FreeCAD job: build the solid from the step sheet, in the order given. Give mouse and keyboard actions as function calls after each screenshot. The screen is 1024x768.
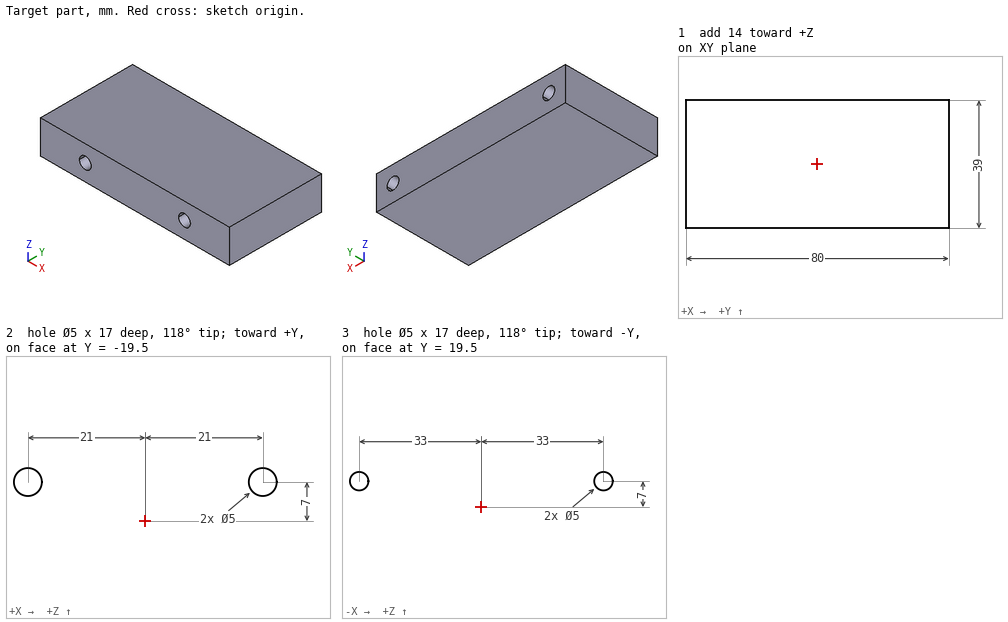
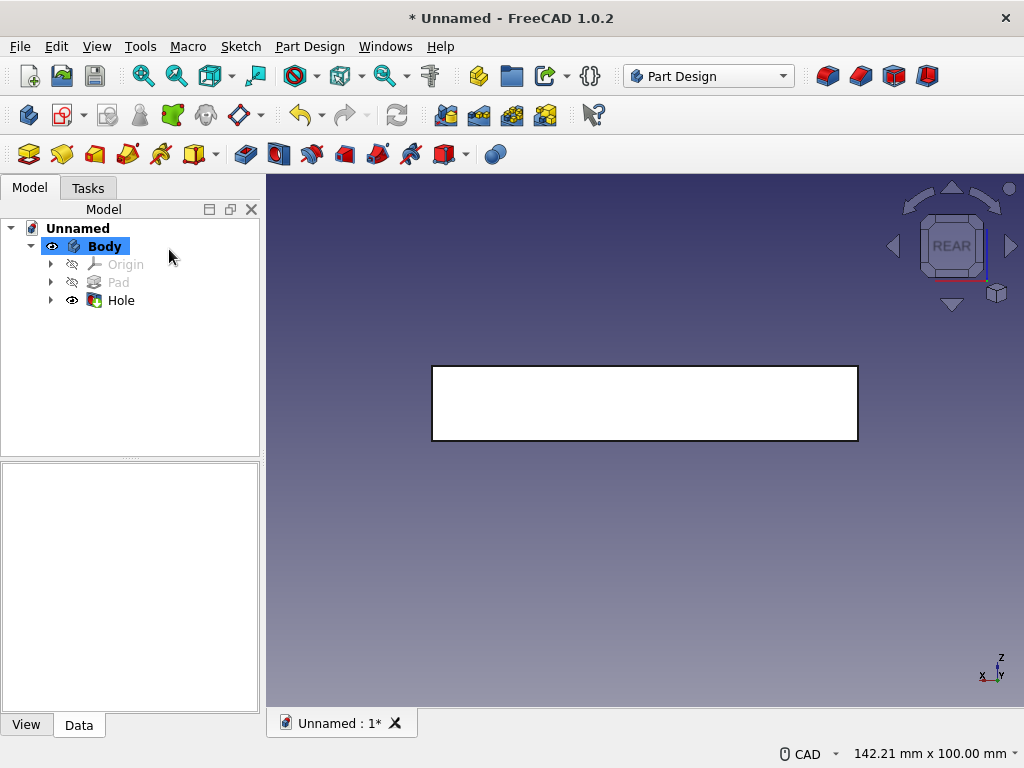
click(523, 402)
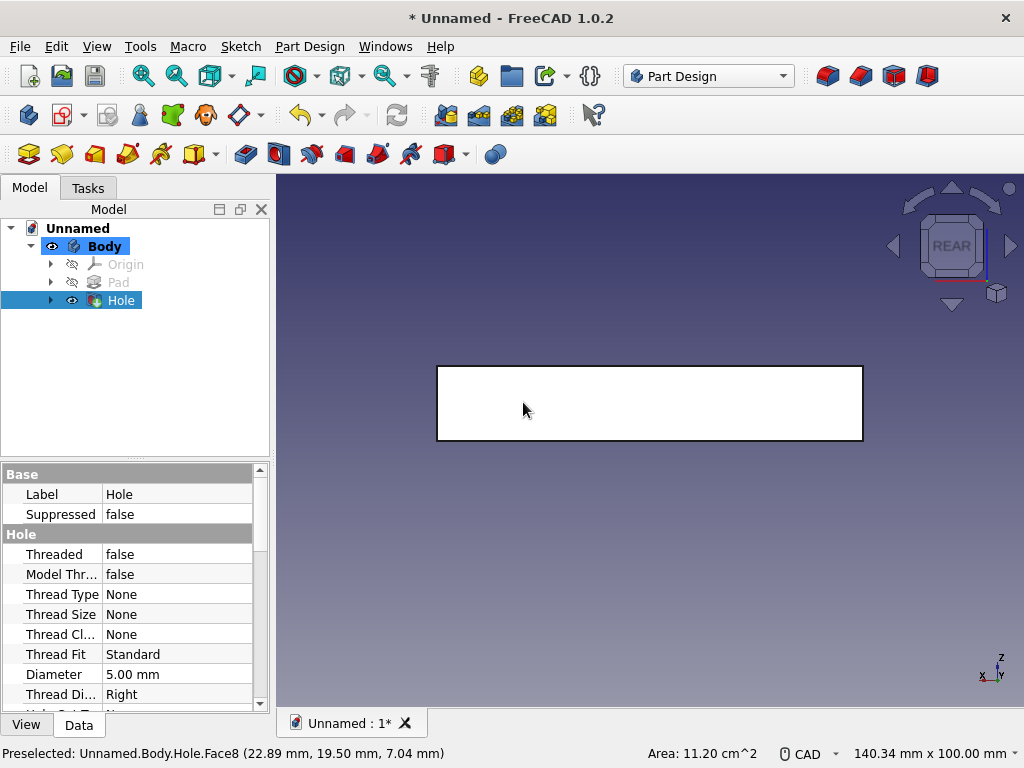
click(62, 116)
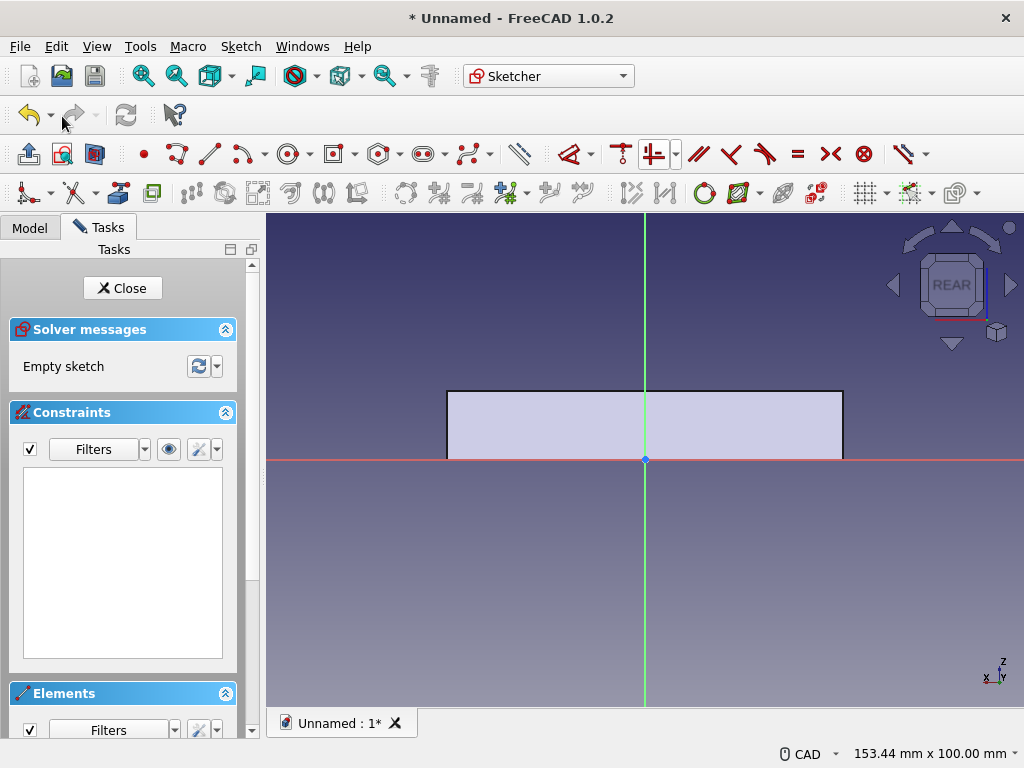
click(288, 154)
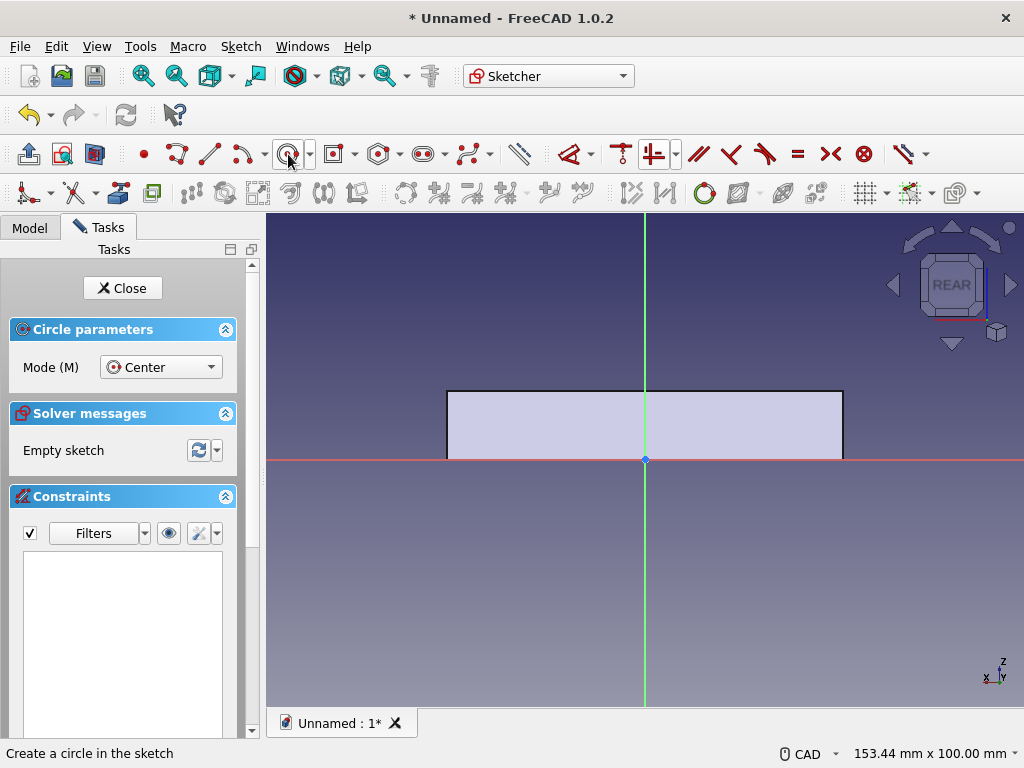
scroll(808, 425, up, 4)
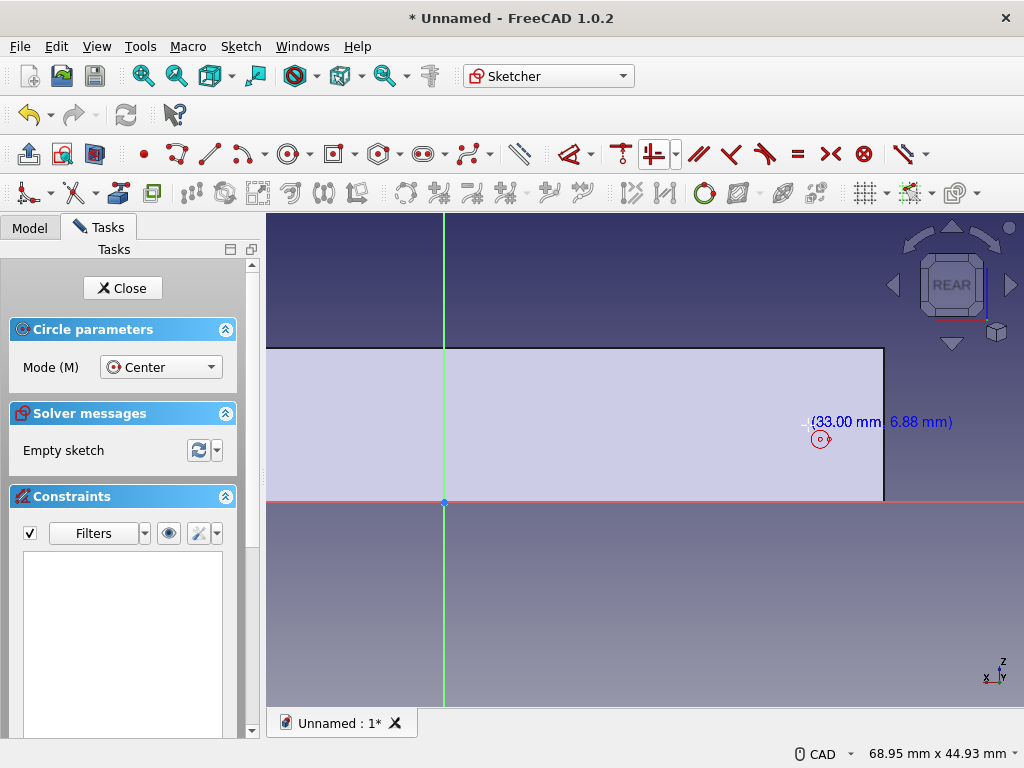
click(807, 425)
move(827, 406)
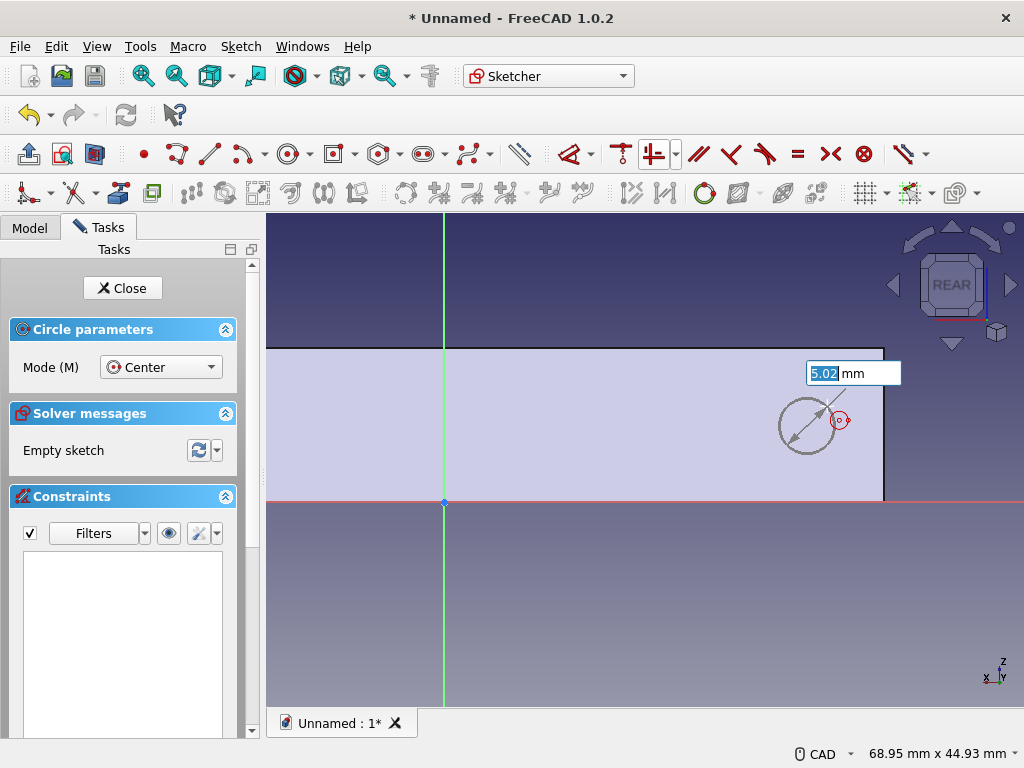
text(5)
key(Return)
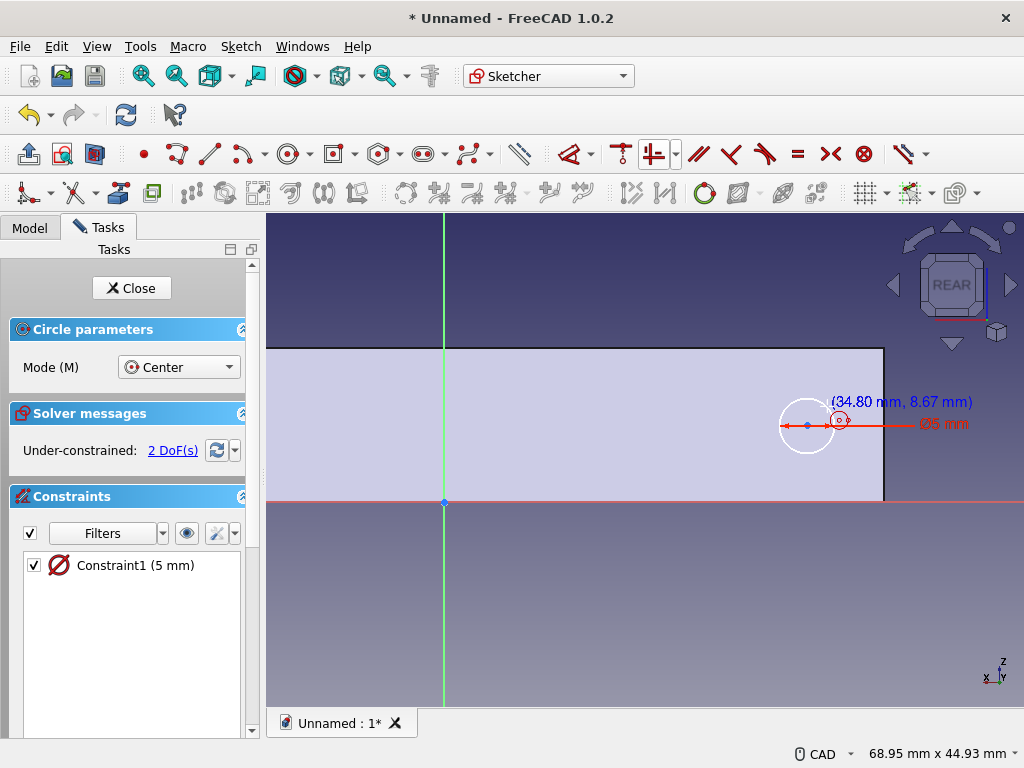
scroll(737, 472, down, 3)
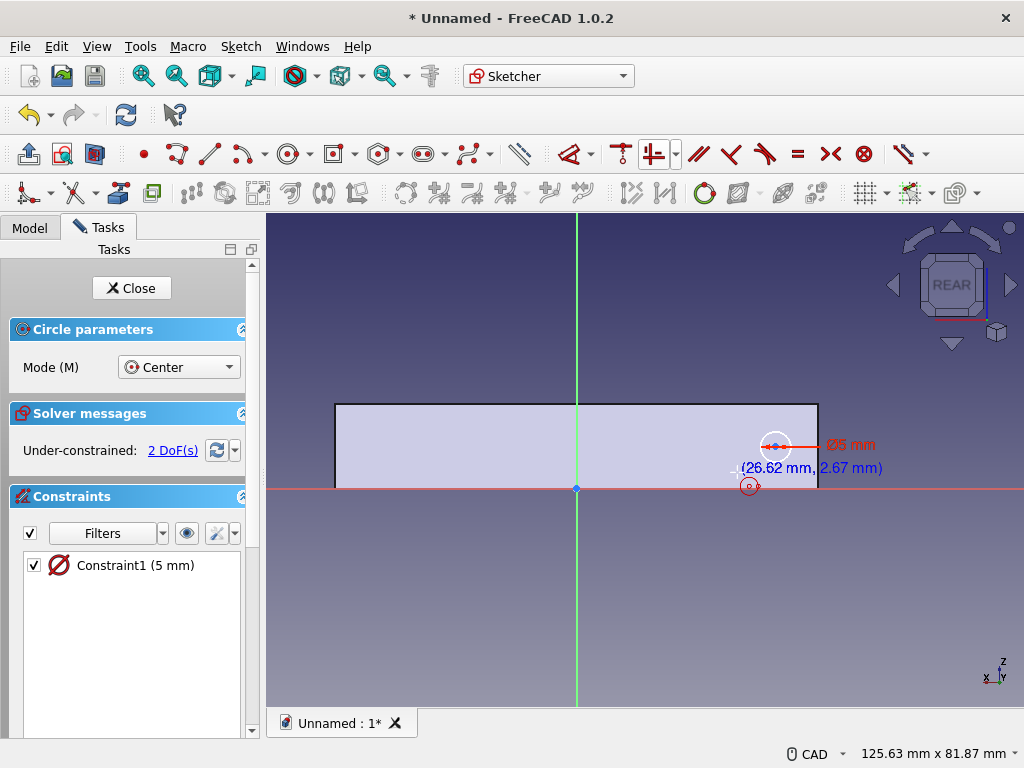
scroll(378, 447, up, 3)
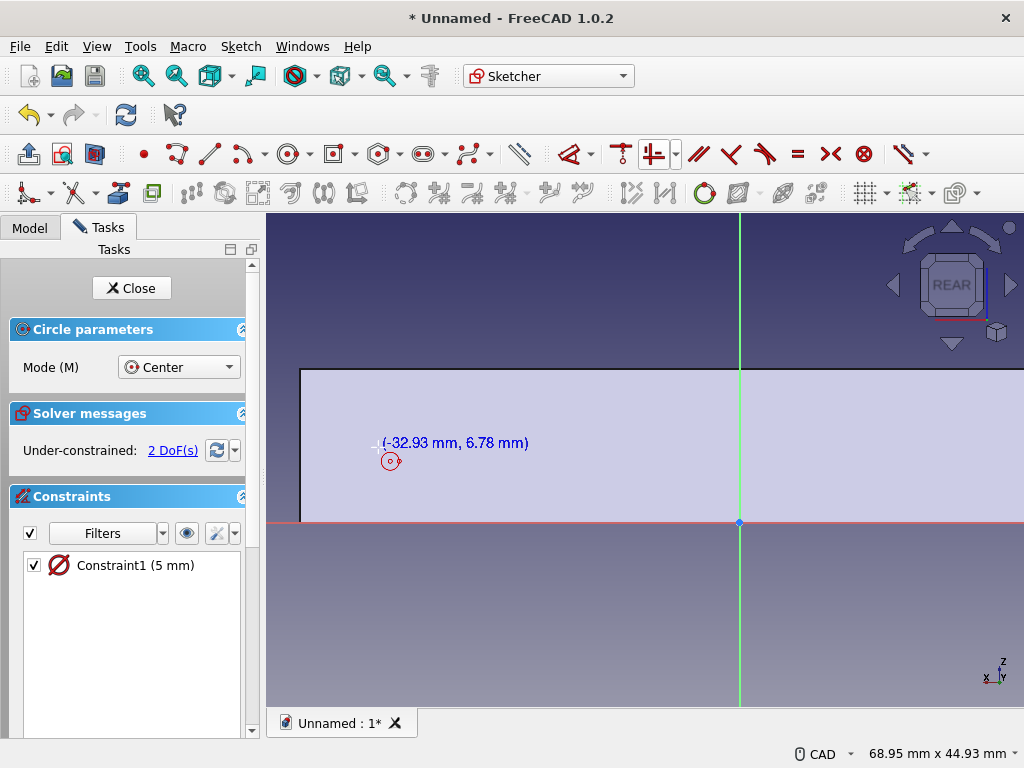
click(377, 446)
move(397, 427)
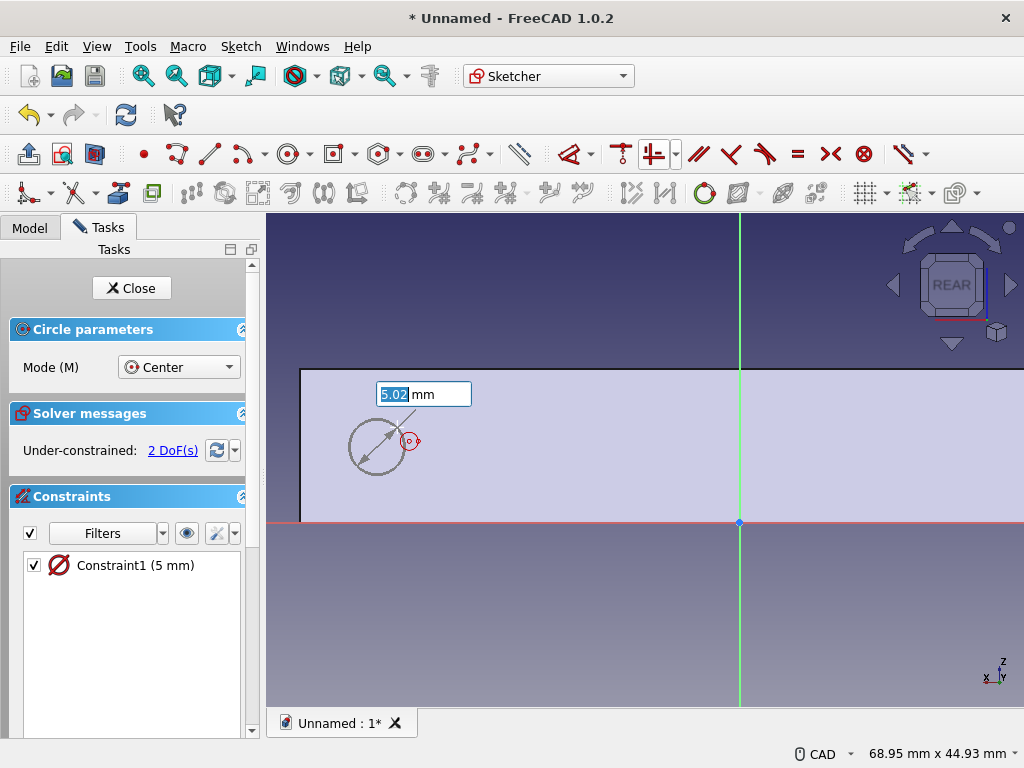
text(5)
key(Return)
key(Escape)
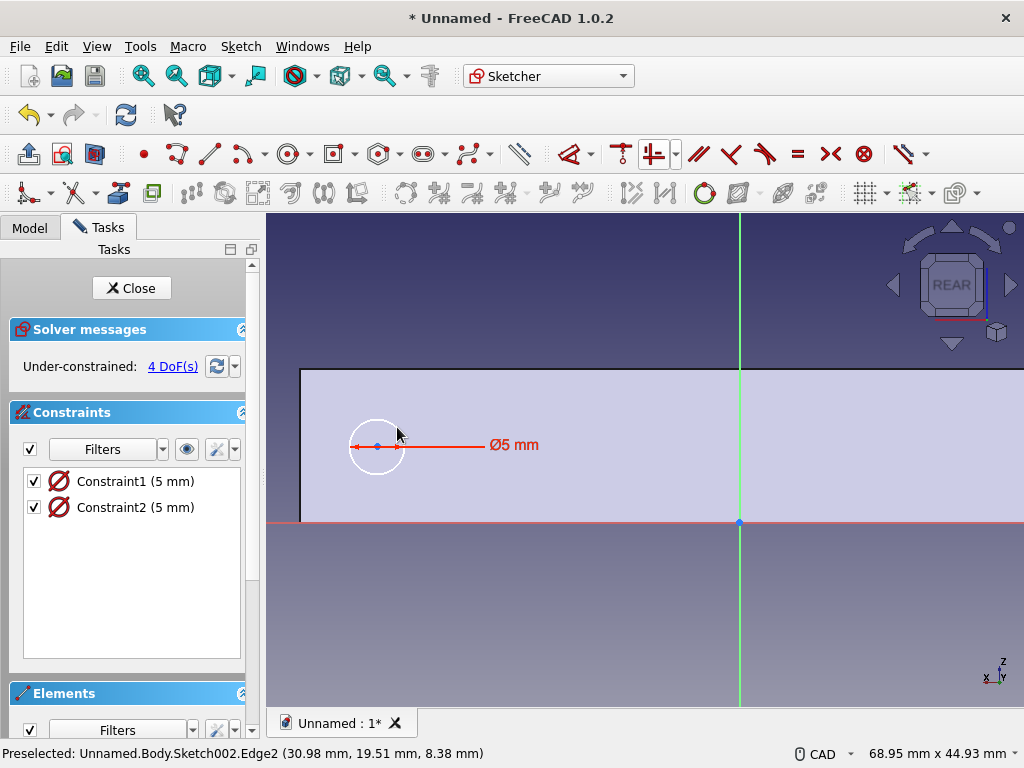
scroll(378, 447, down, 3)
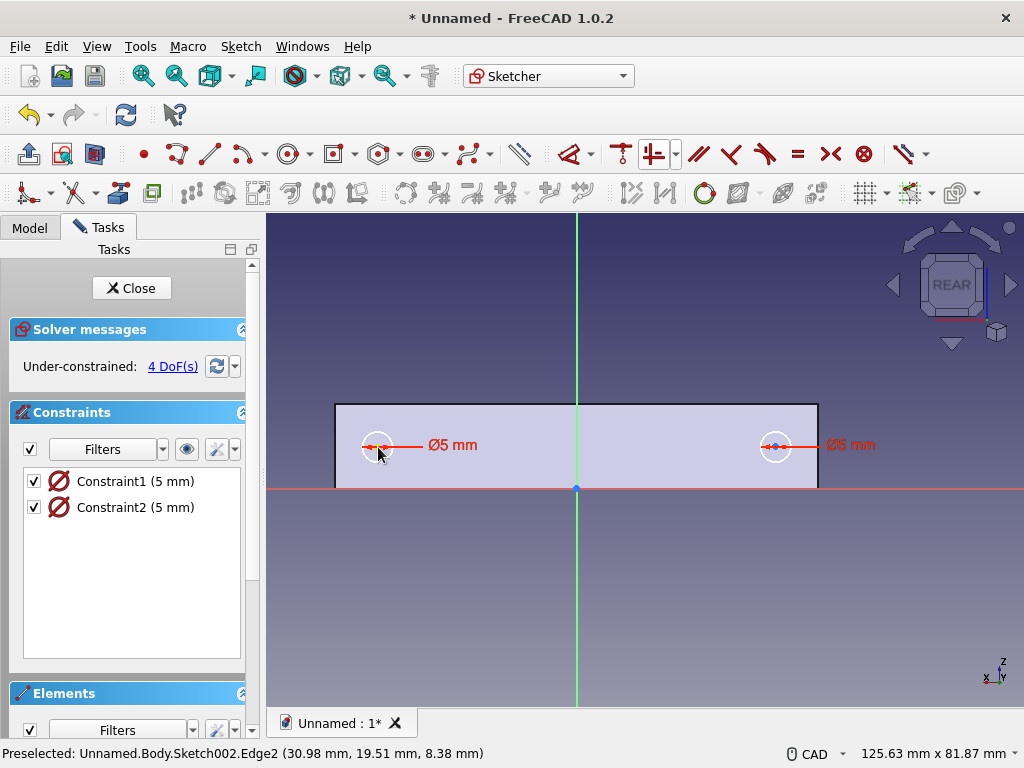
click(776, 447)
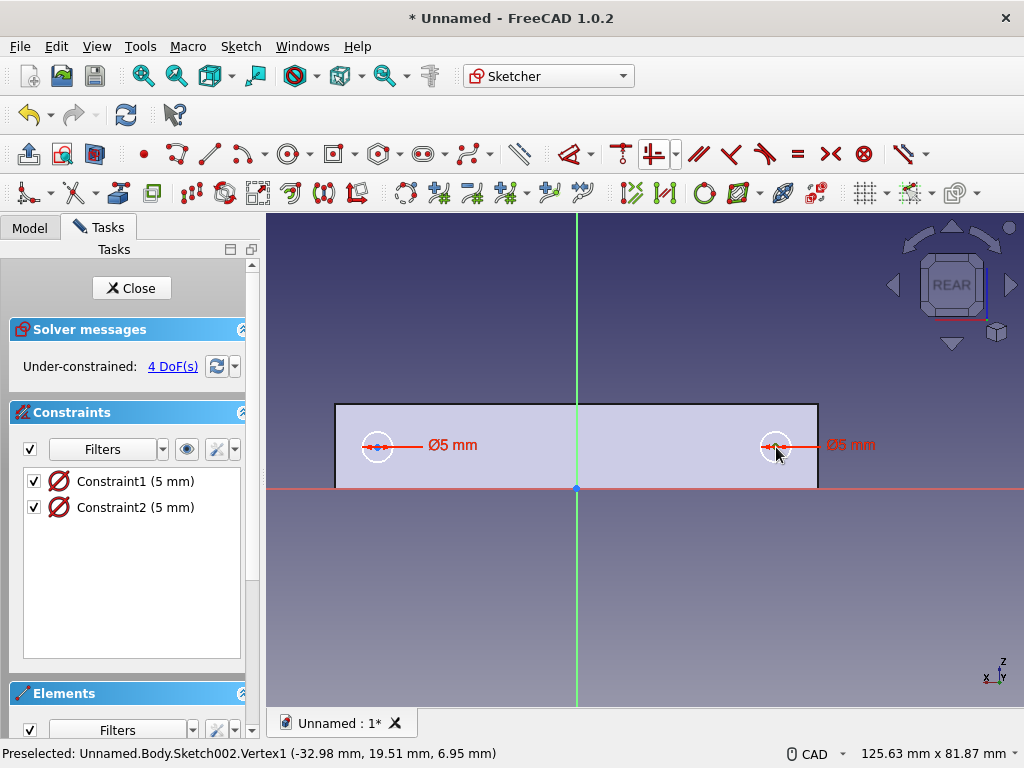
click(378, 447)